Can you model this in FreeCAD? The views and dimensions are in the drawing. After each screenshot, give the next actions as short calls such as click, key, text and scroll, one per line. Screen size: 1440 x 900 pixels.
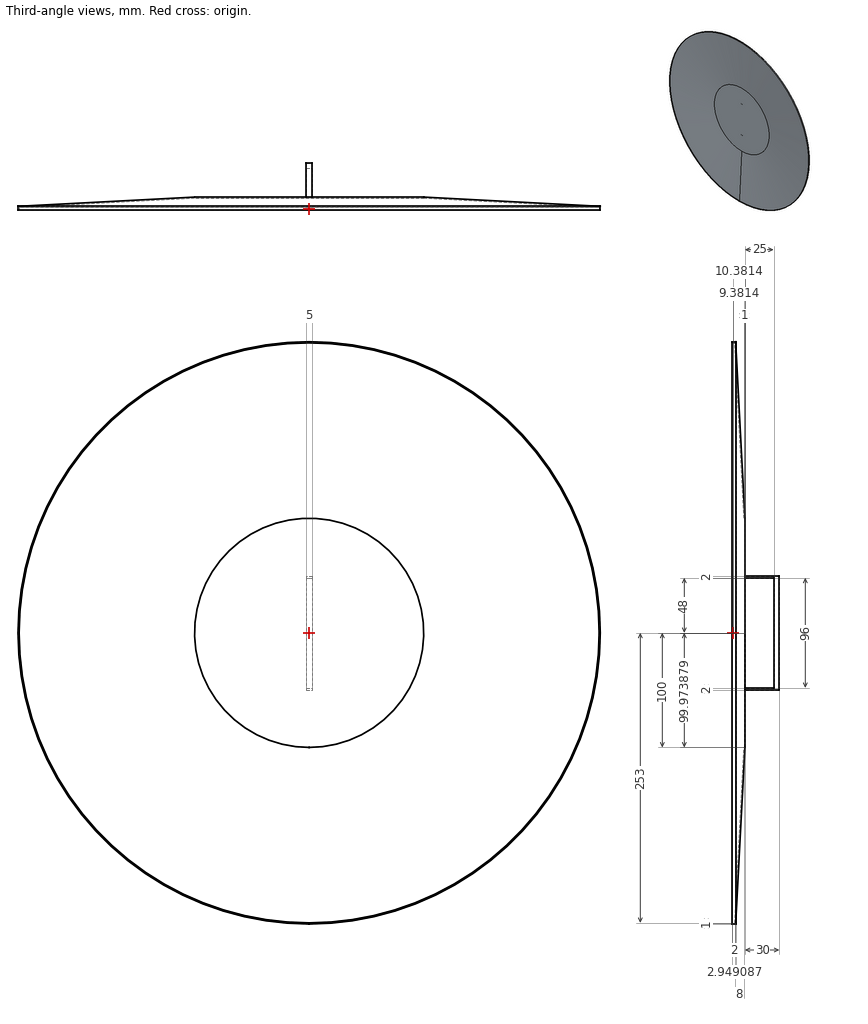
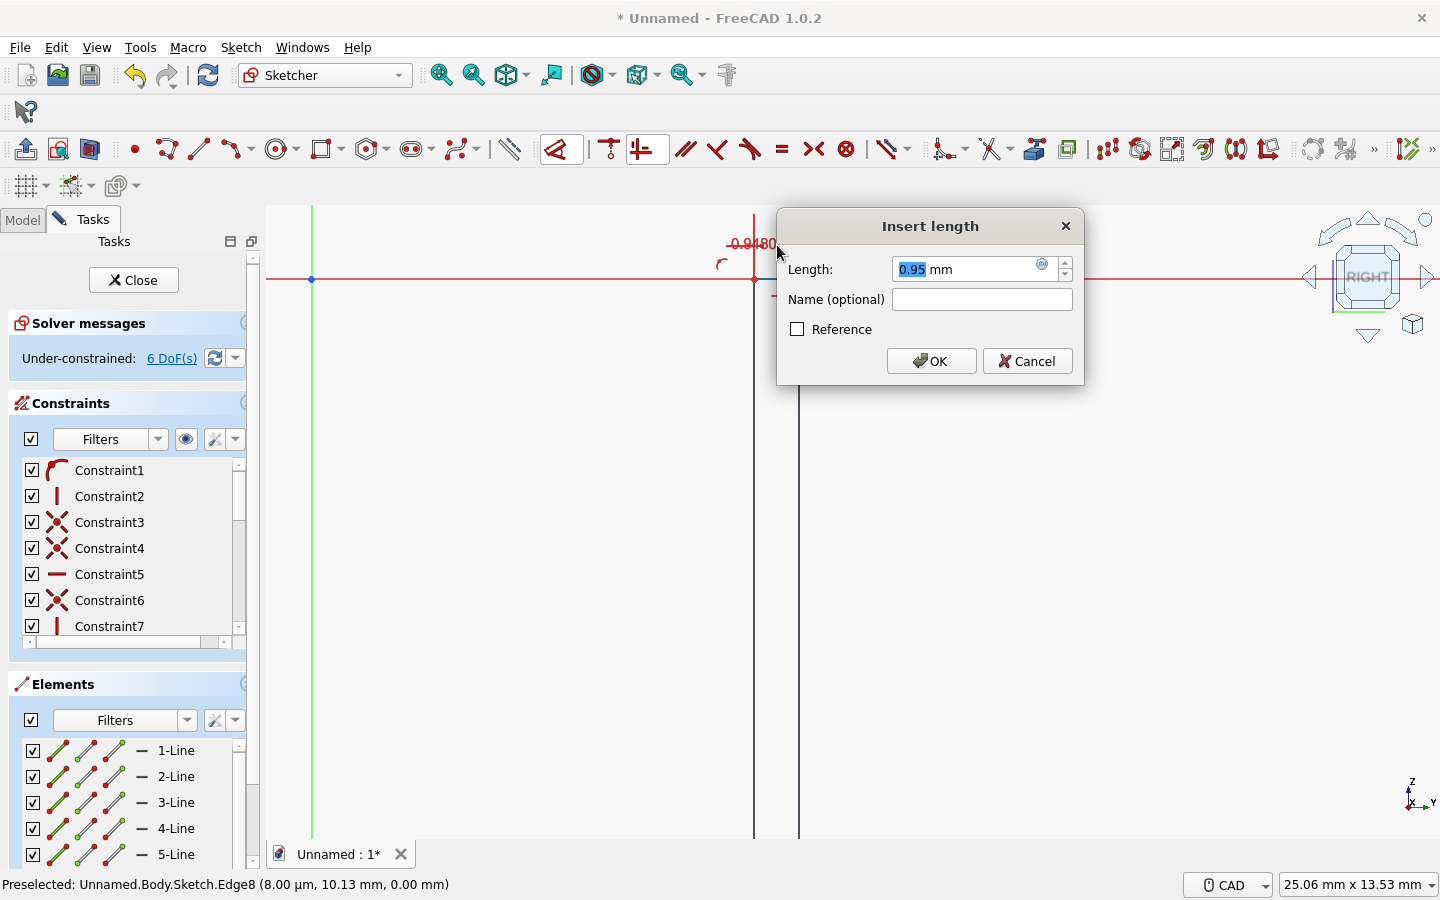
text(1)
key(Return)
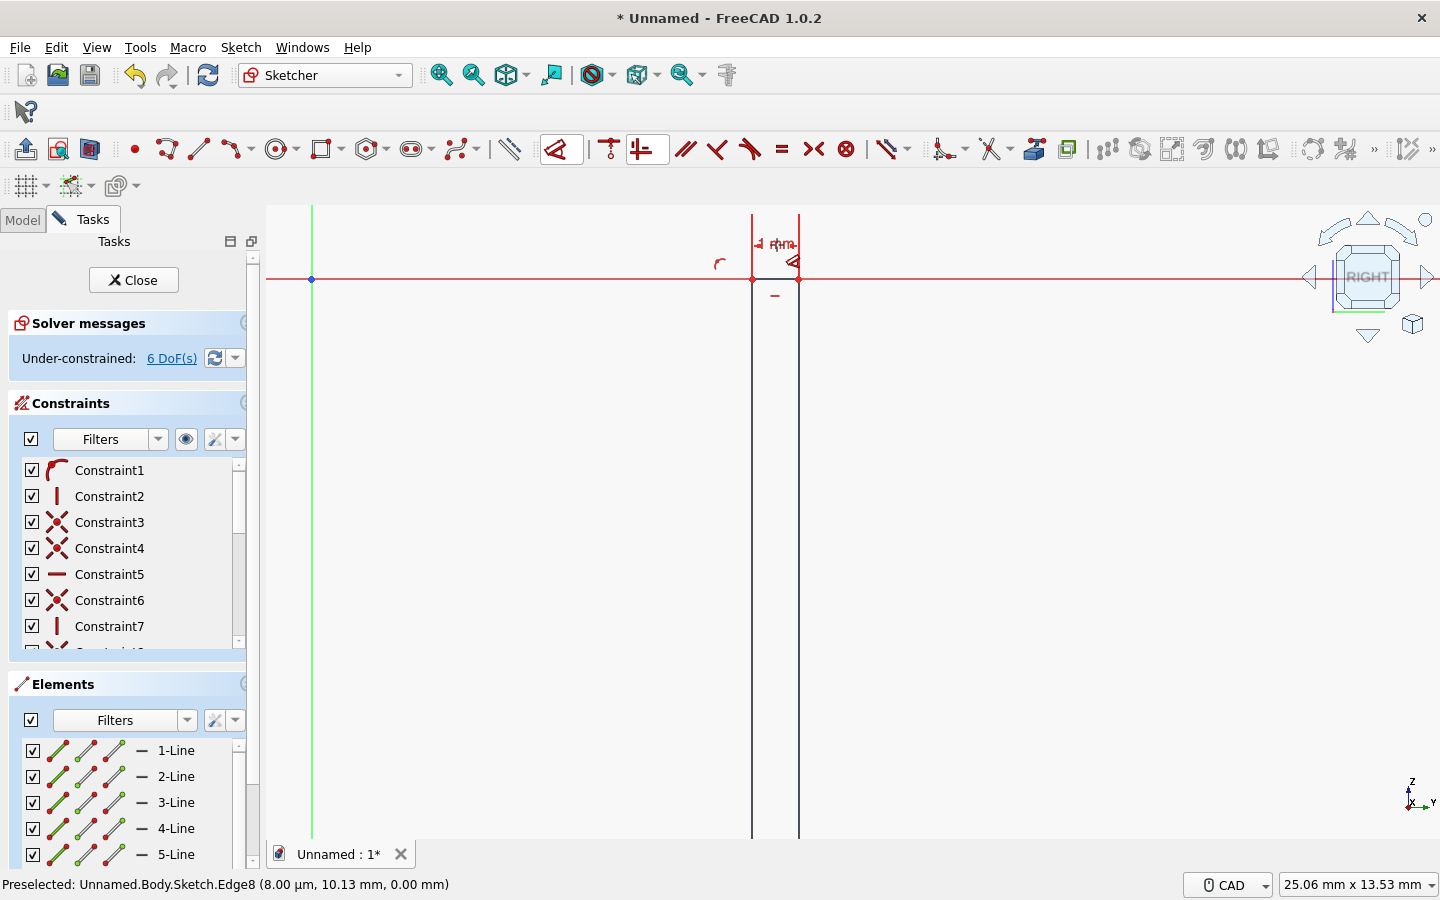
scroll(795, 279, down, 16)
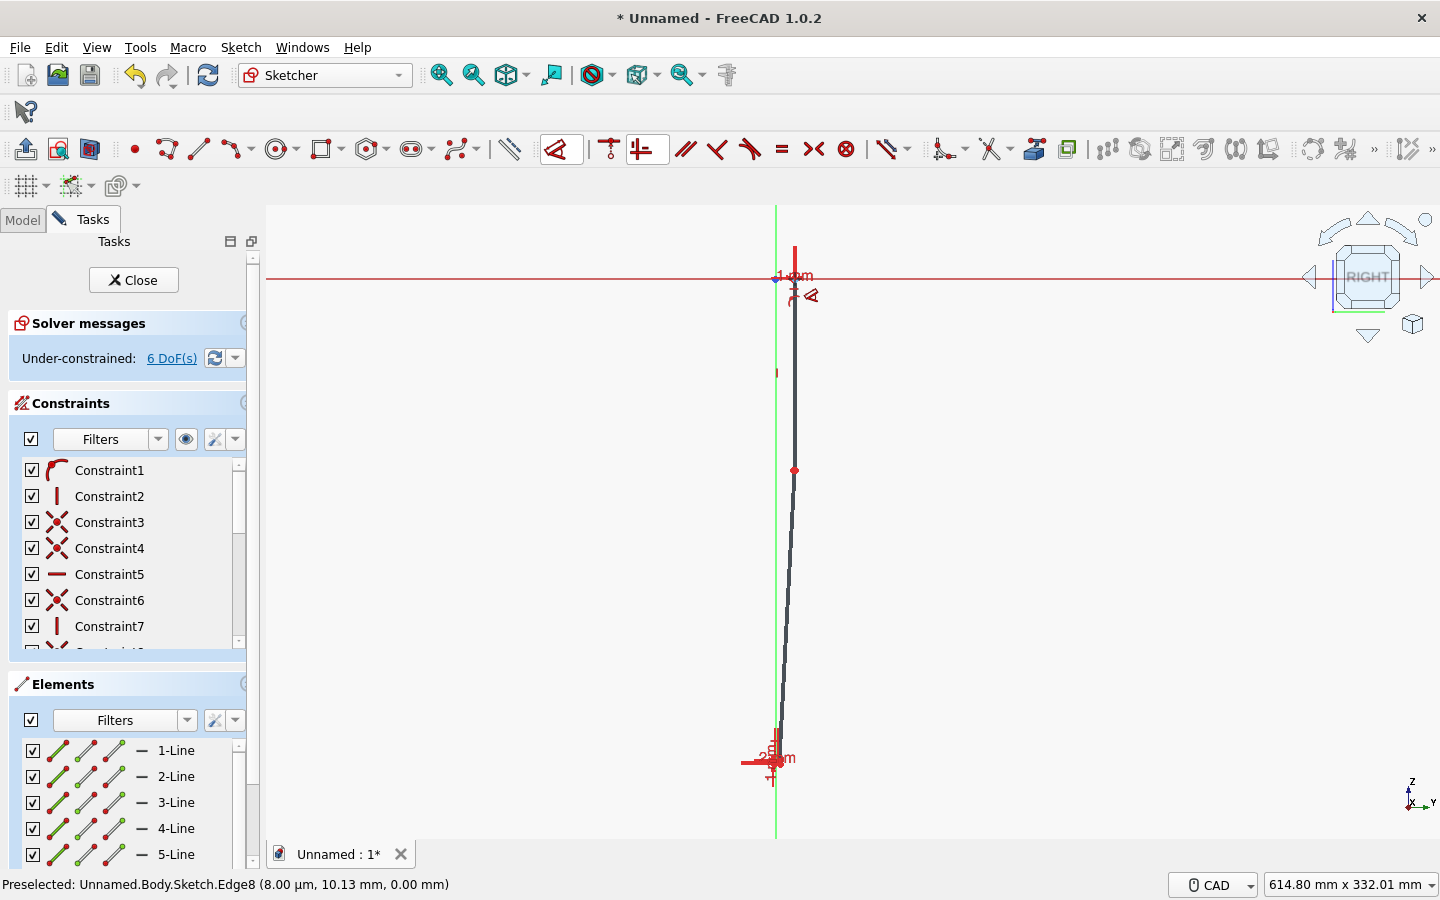
scroll(789, 558, up, 10)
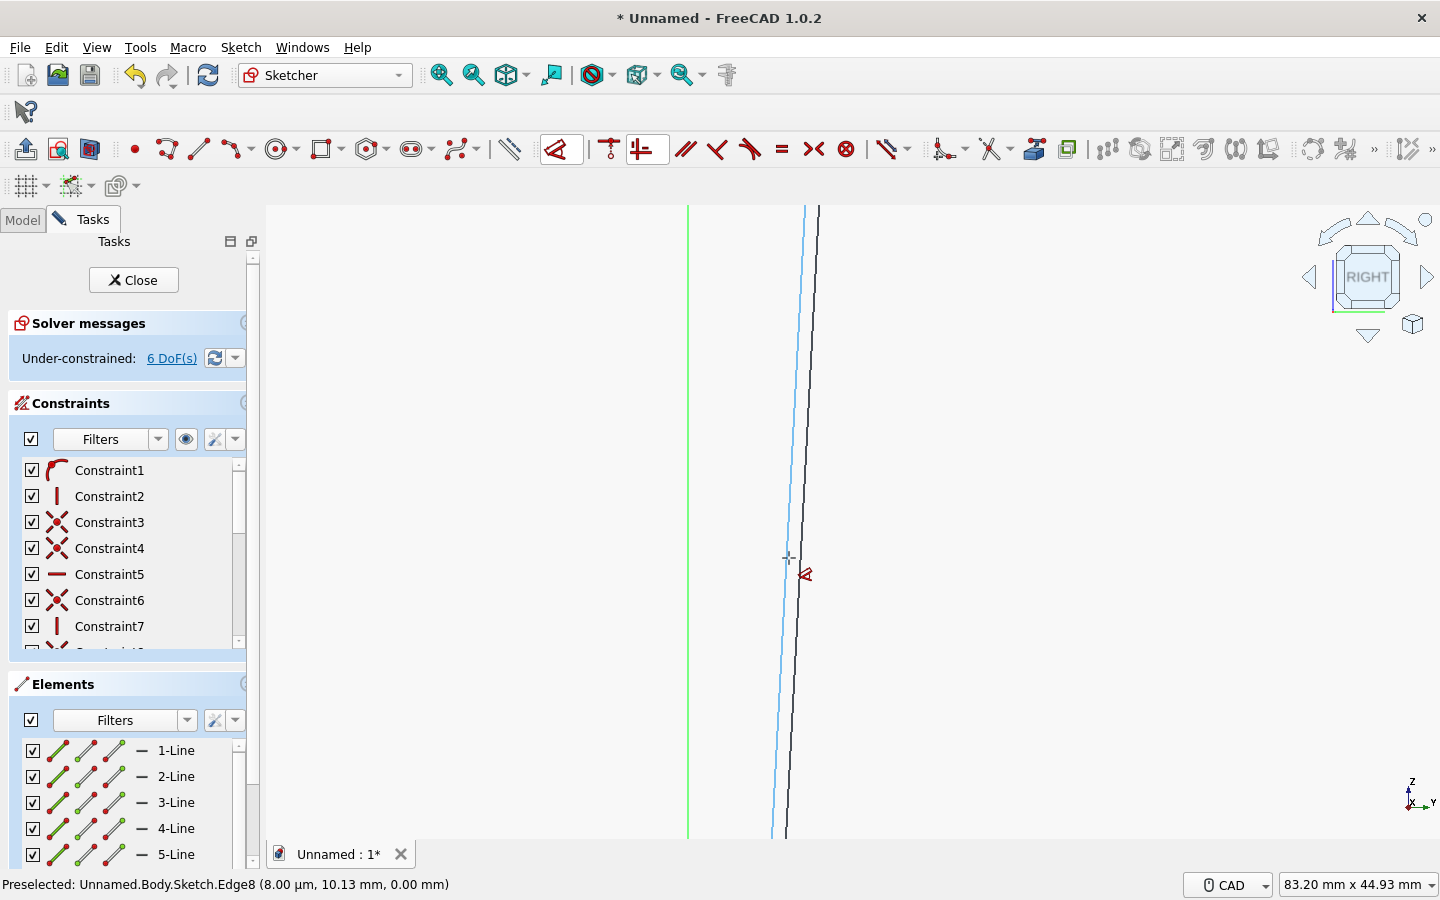
click(787, 556)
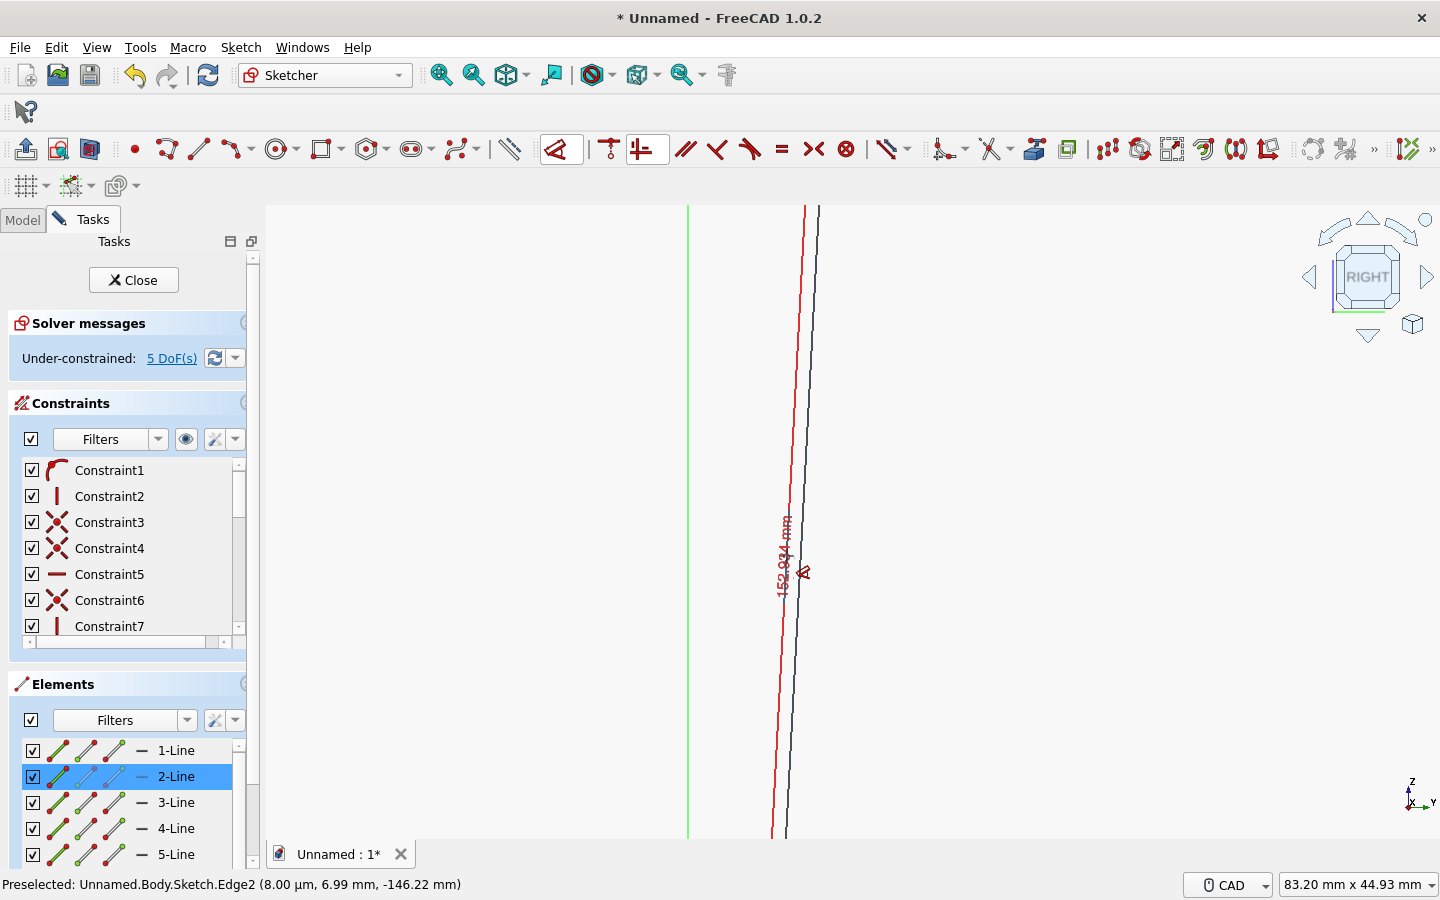
key(Escape)
key(Escape)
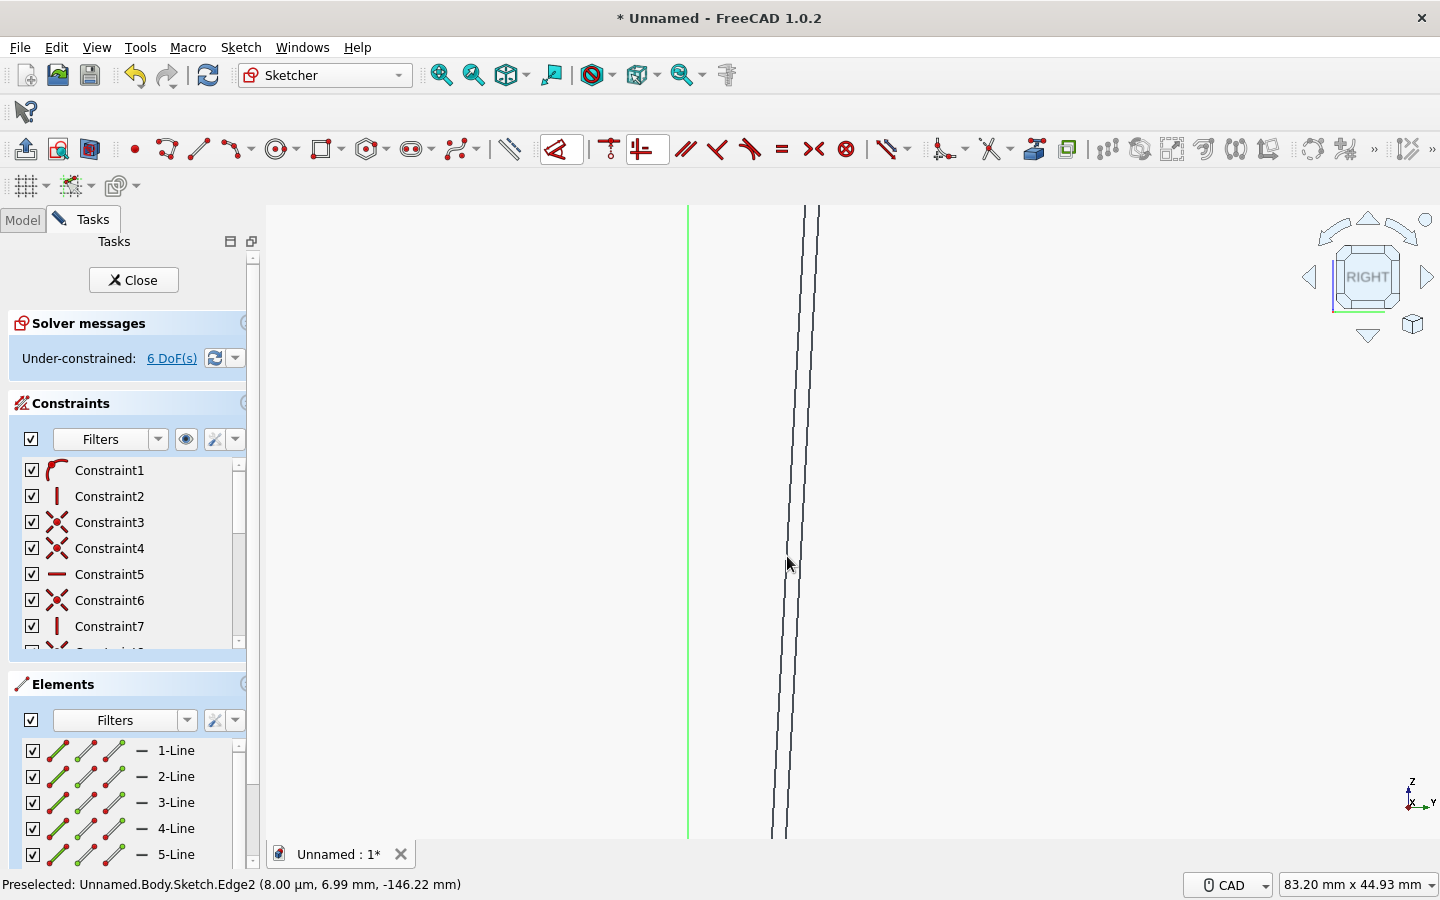
click(787, 556)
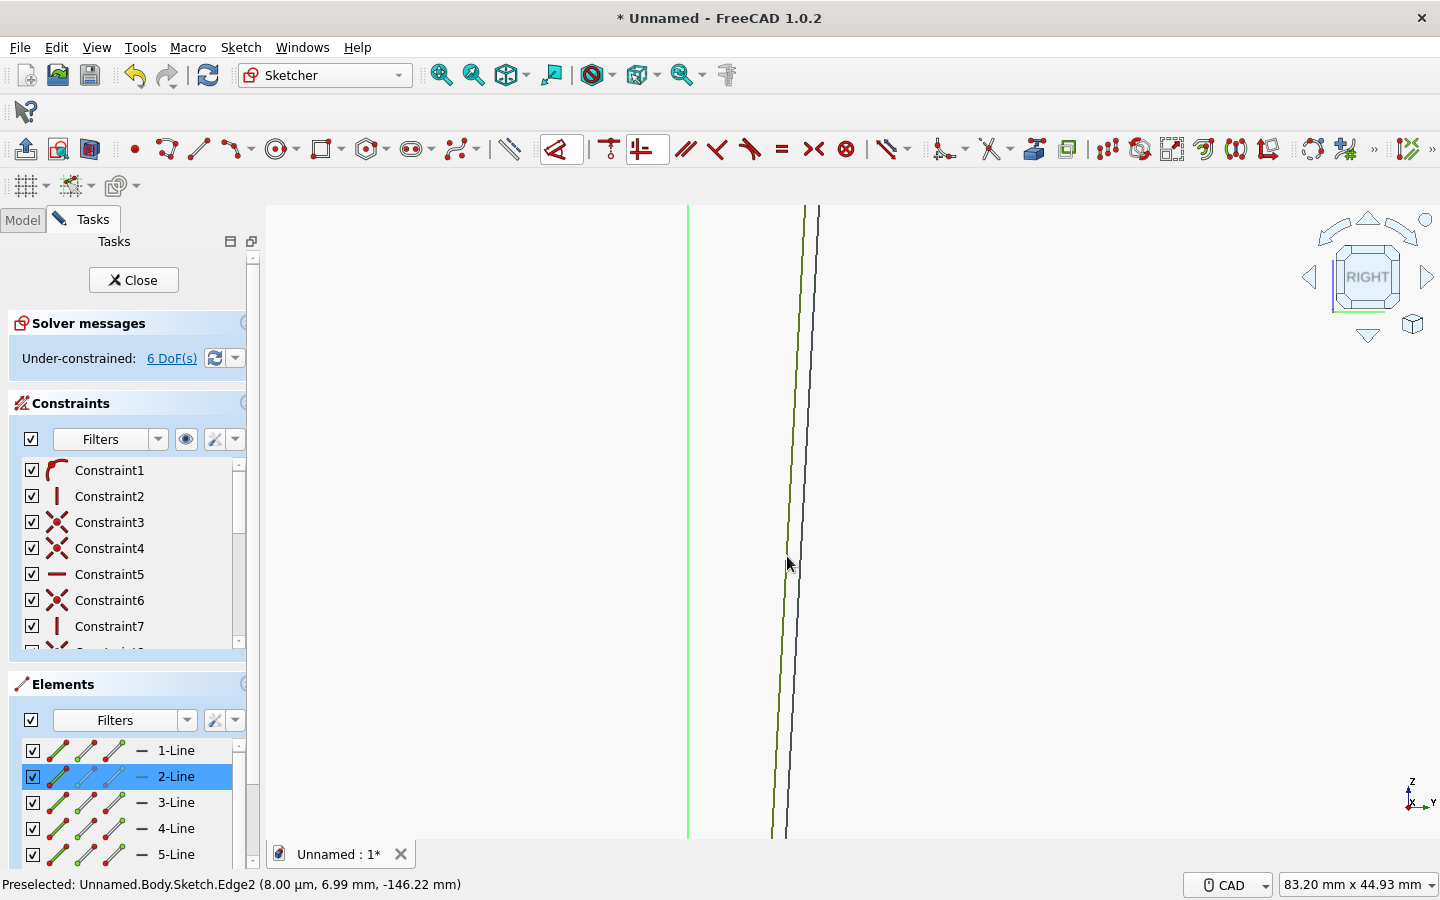
key(l)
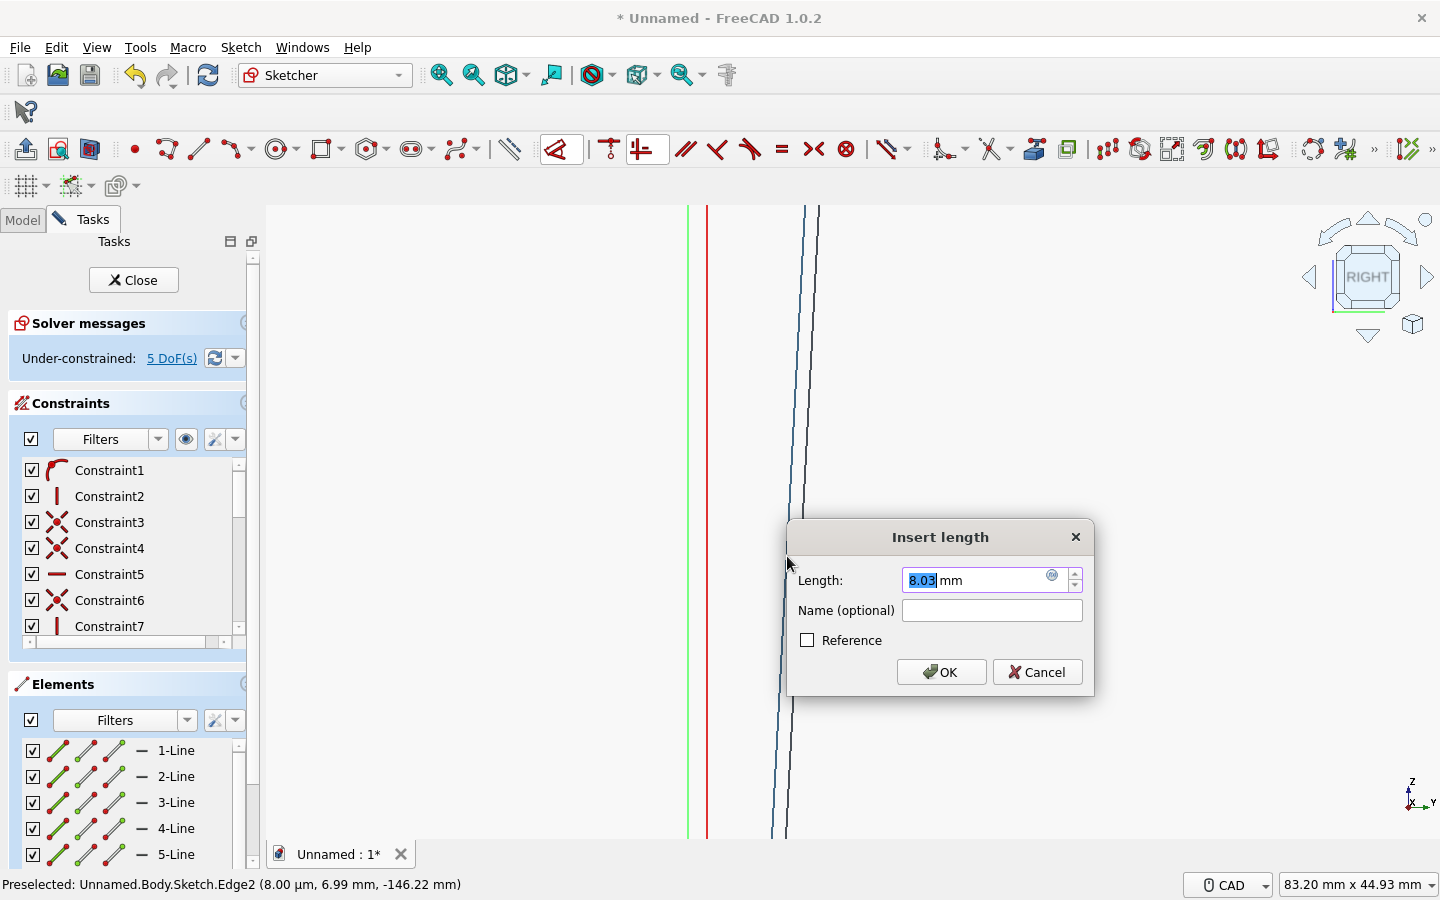
text(8)
key(Return)